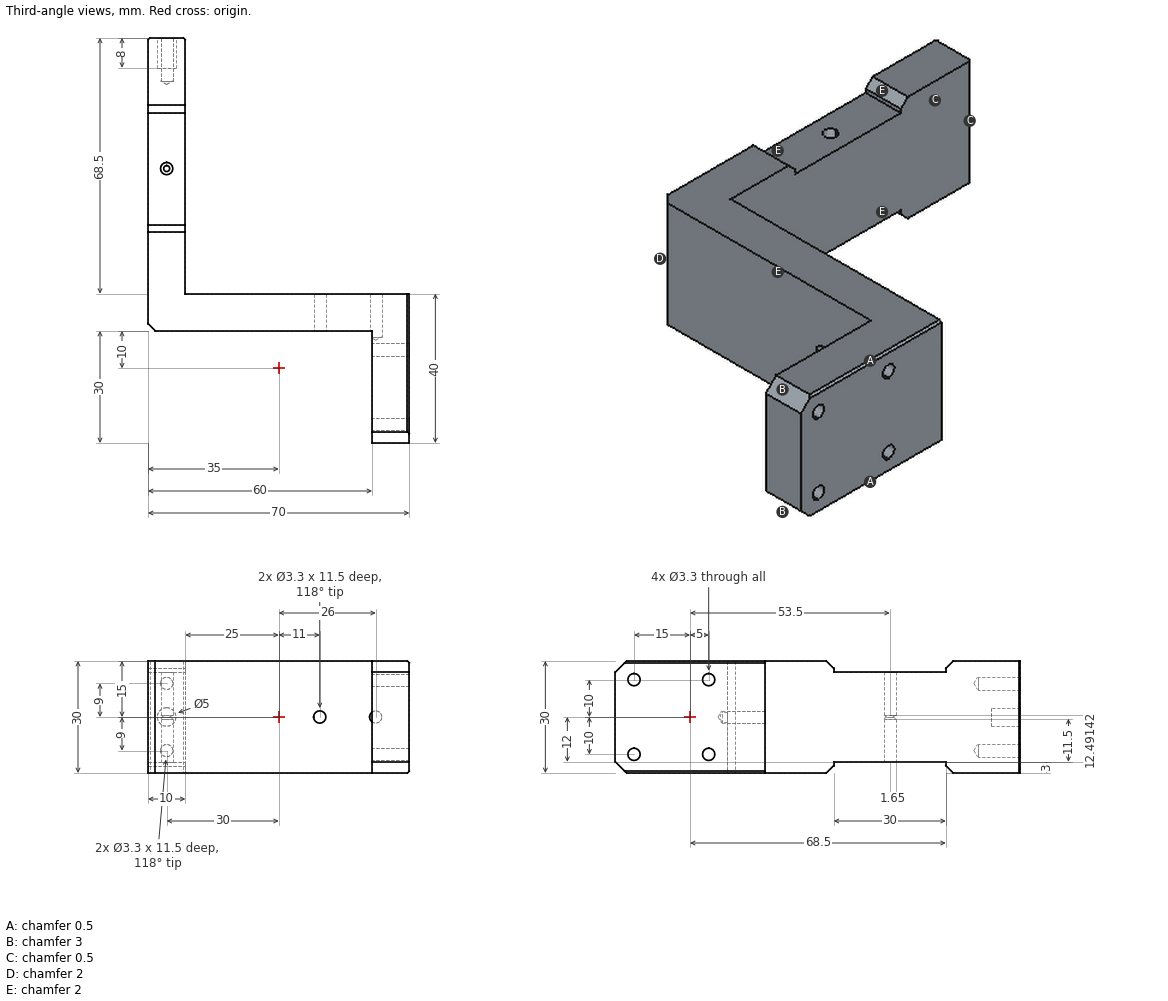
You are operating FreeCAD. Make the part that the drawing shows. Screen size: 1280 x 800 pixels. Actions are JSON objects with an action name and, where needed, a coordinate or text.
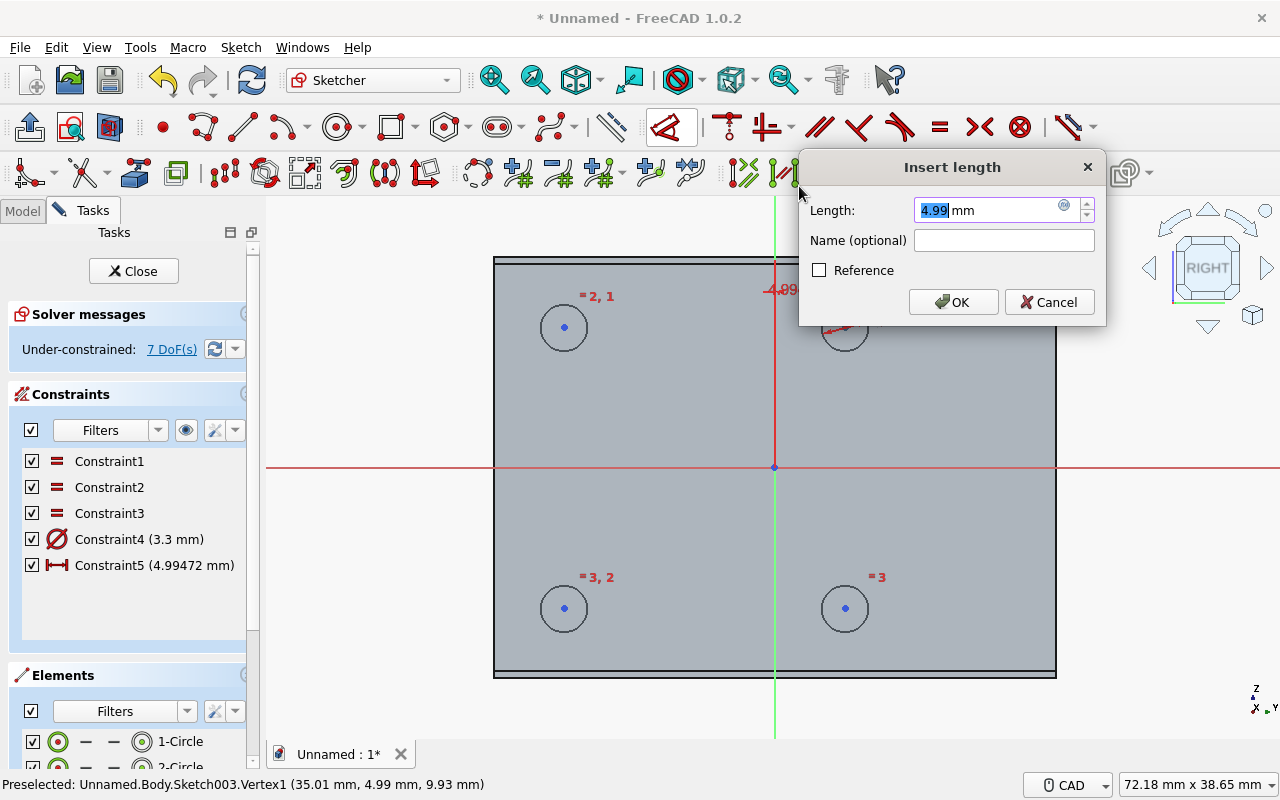
{"action": "type", "text": "5"}
{"action": "key", "text": "Return"}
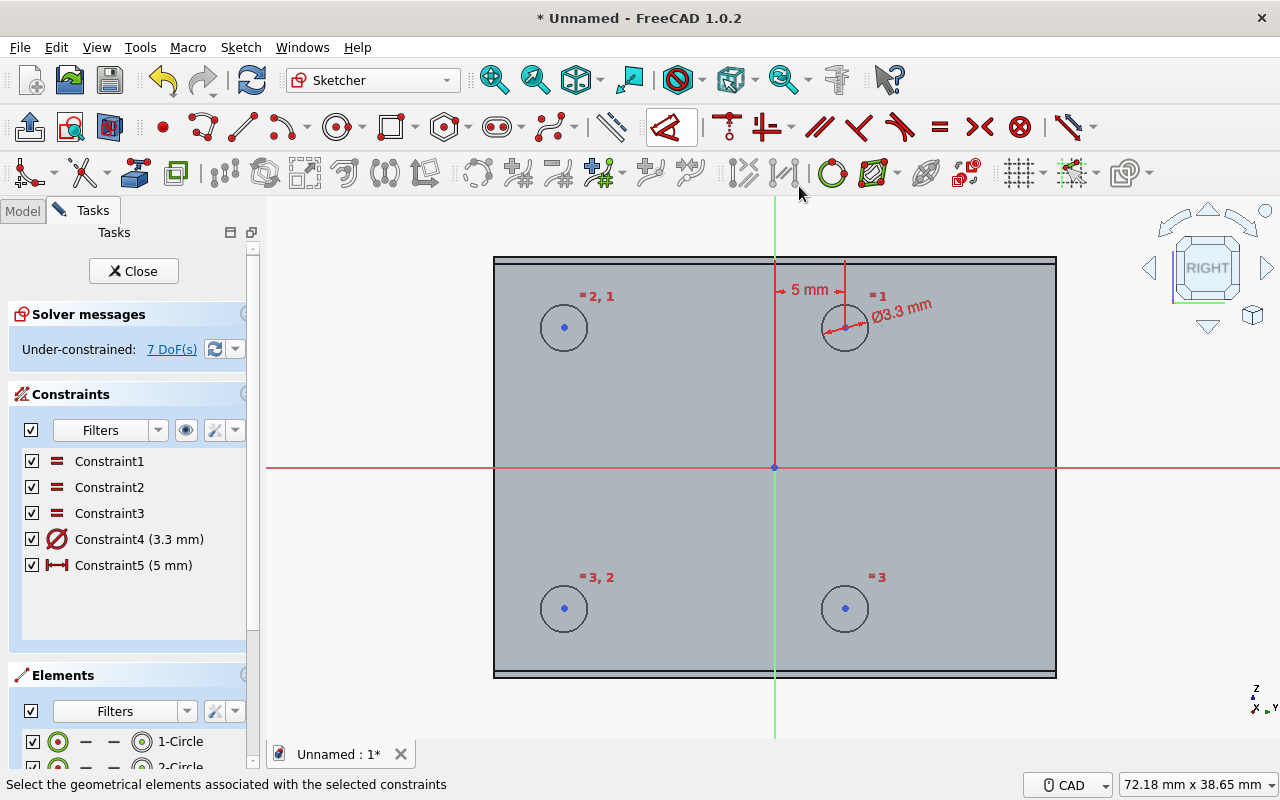
{"action": "left_click", "coordinate": [845, 609]}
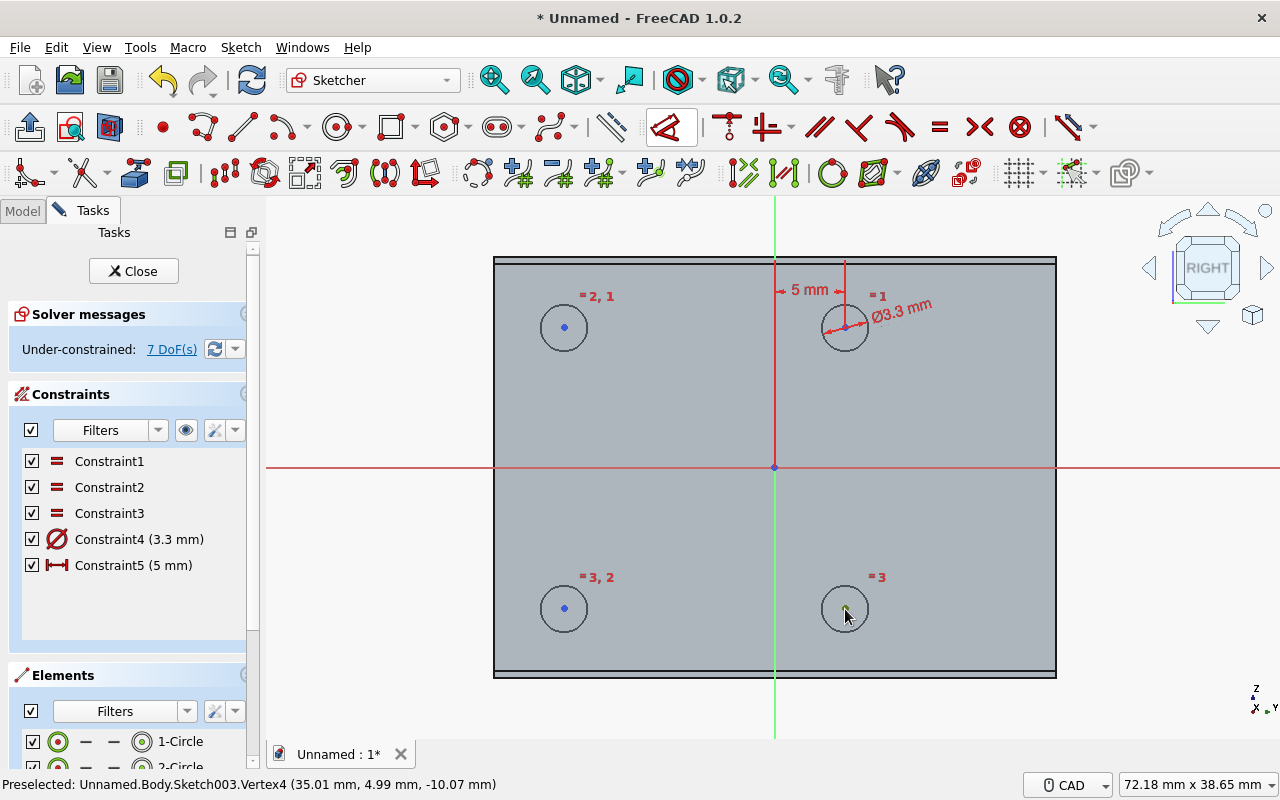
{"action": "left_click", "coordinate": [692, 128]}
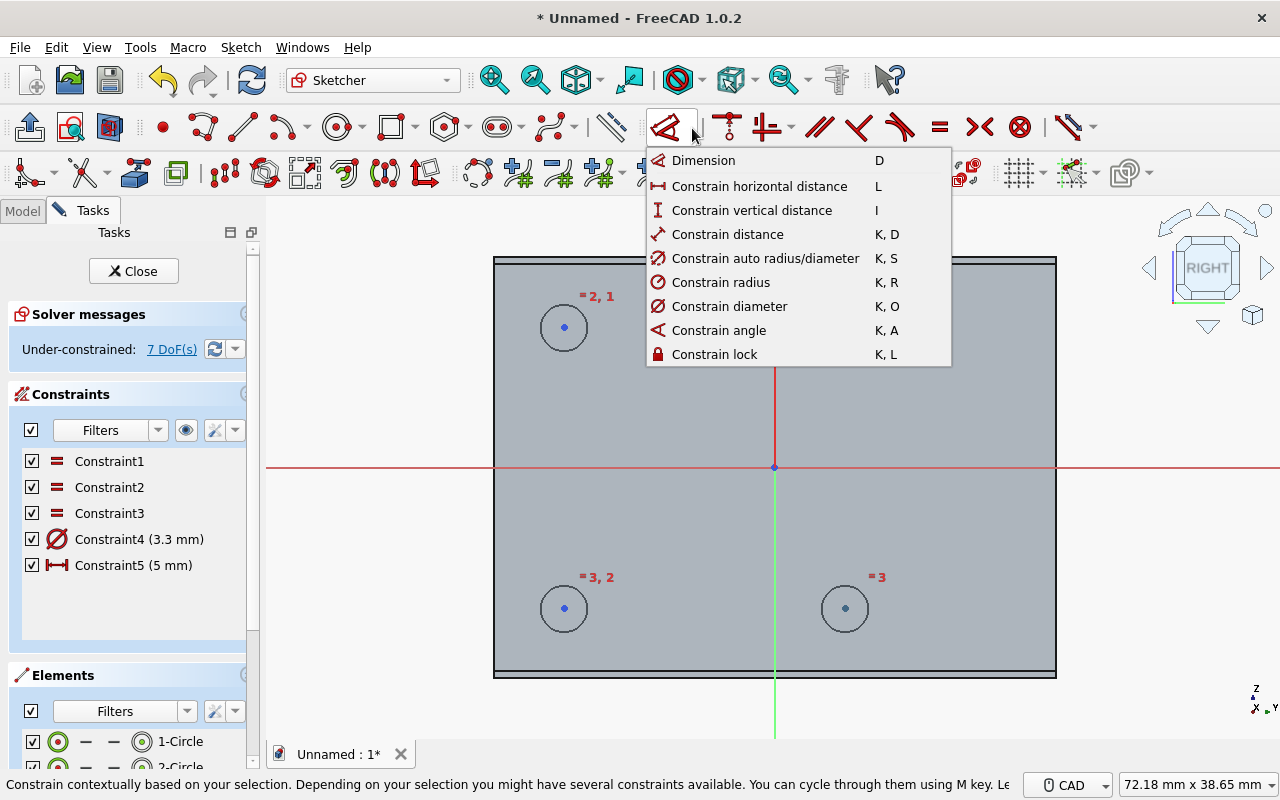
{"action": "left_click", "coordinate": [799, 186]}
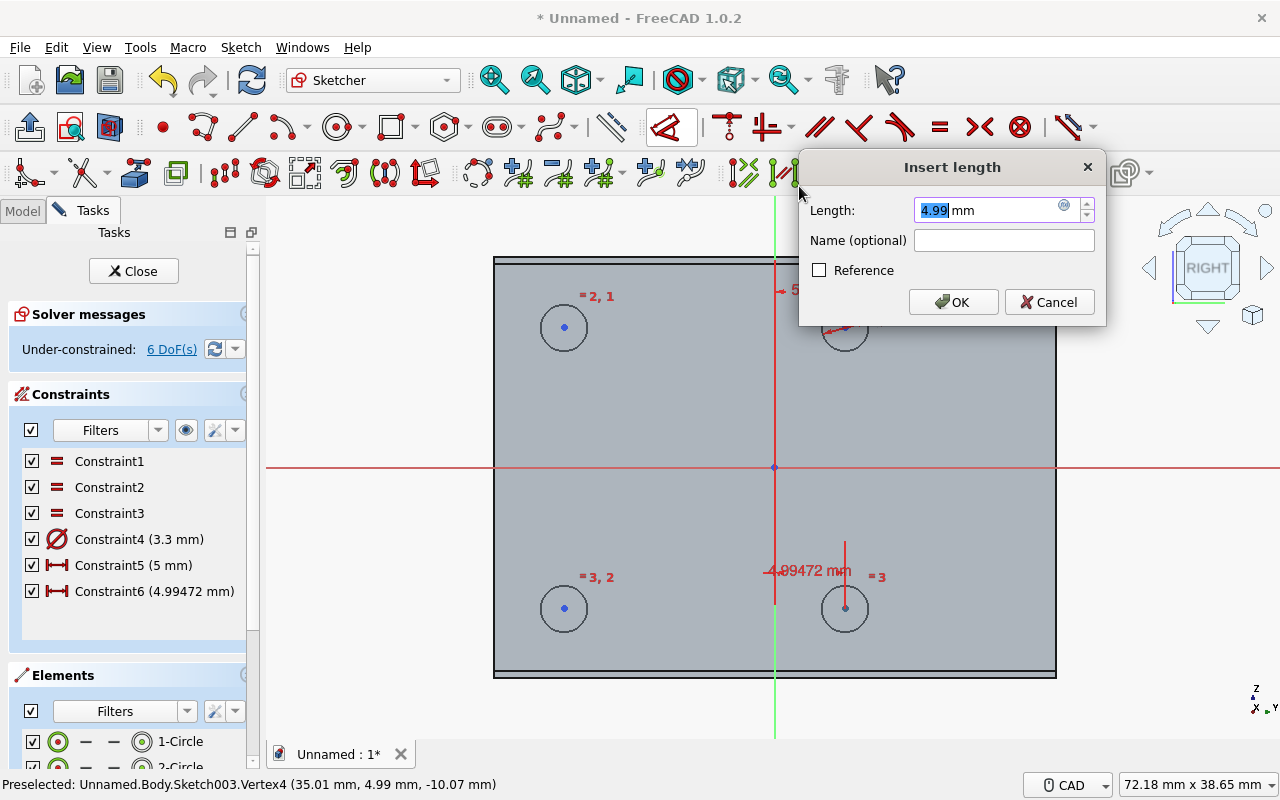
{"action": "type", "text": "5"}
{"action": "key", "text": "Return"}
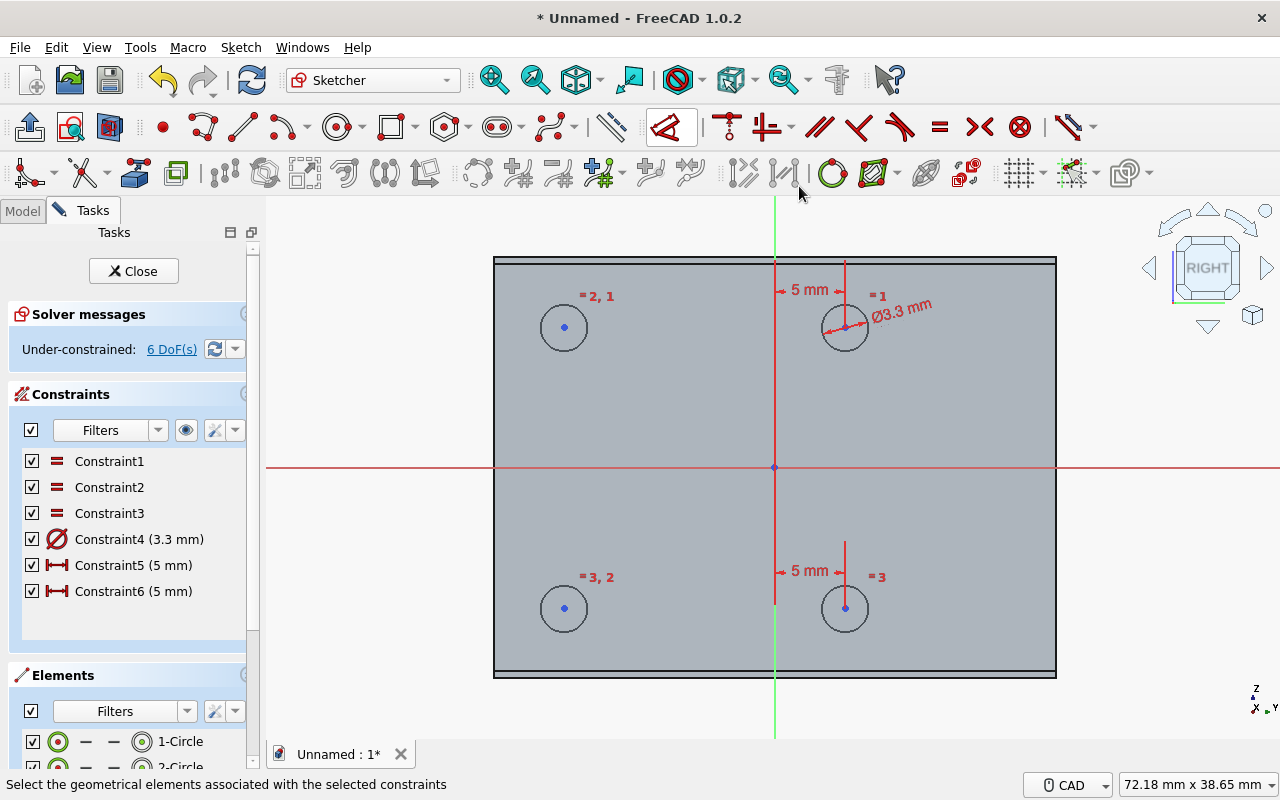
{"action": "left_click", "coordinate": [845, 328]}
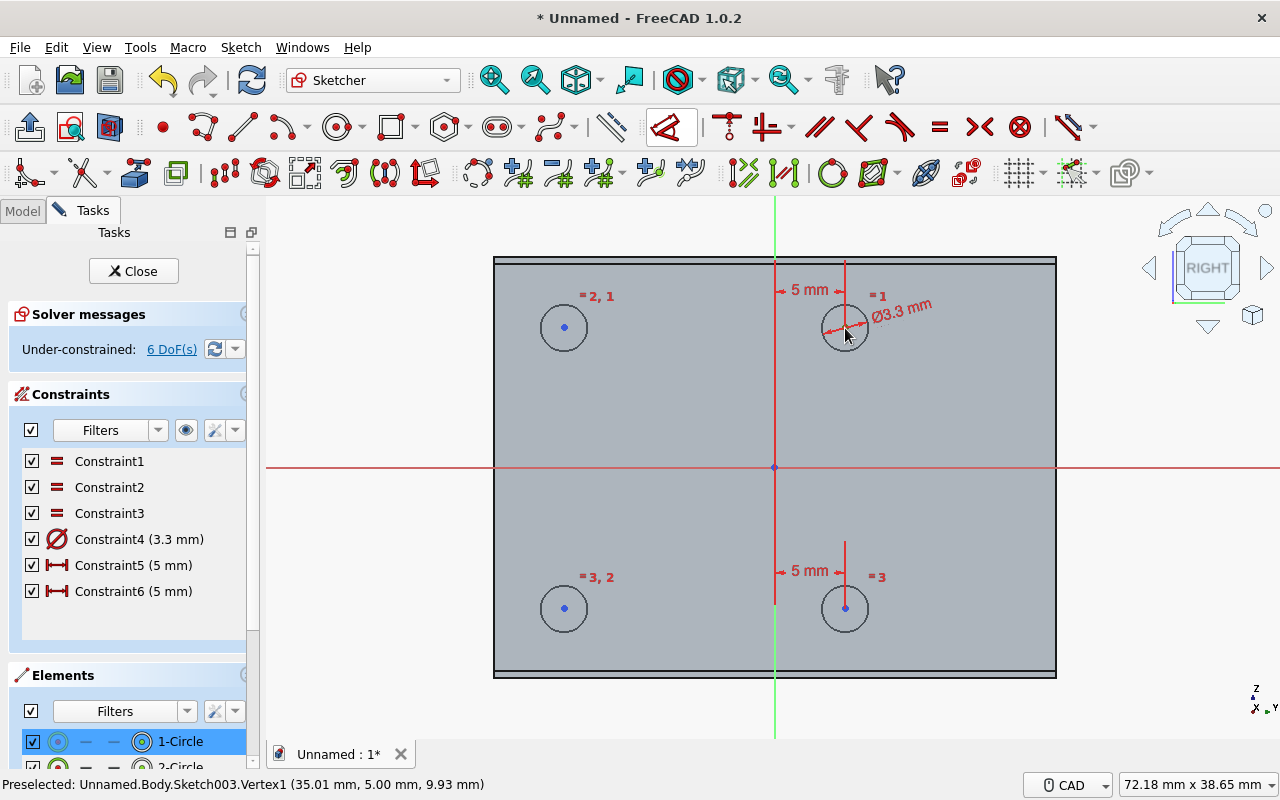
{"action": "key", "text": "i"}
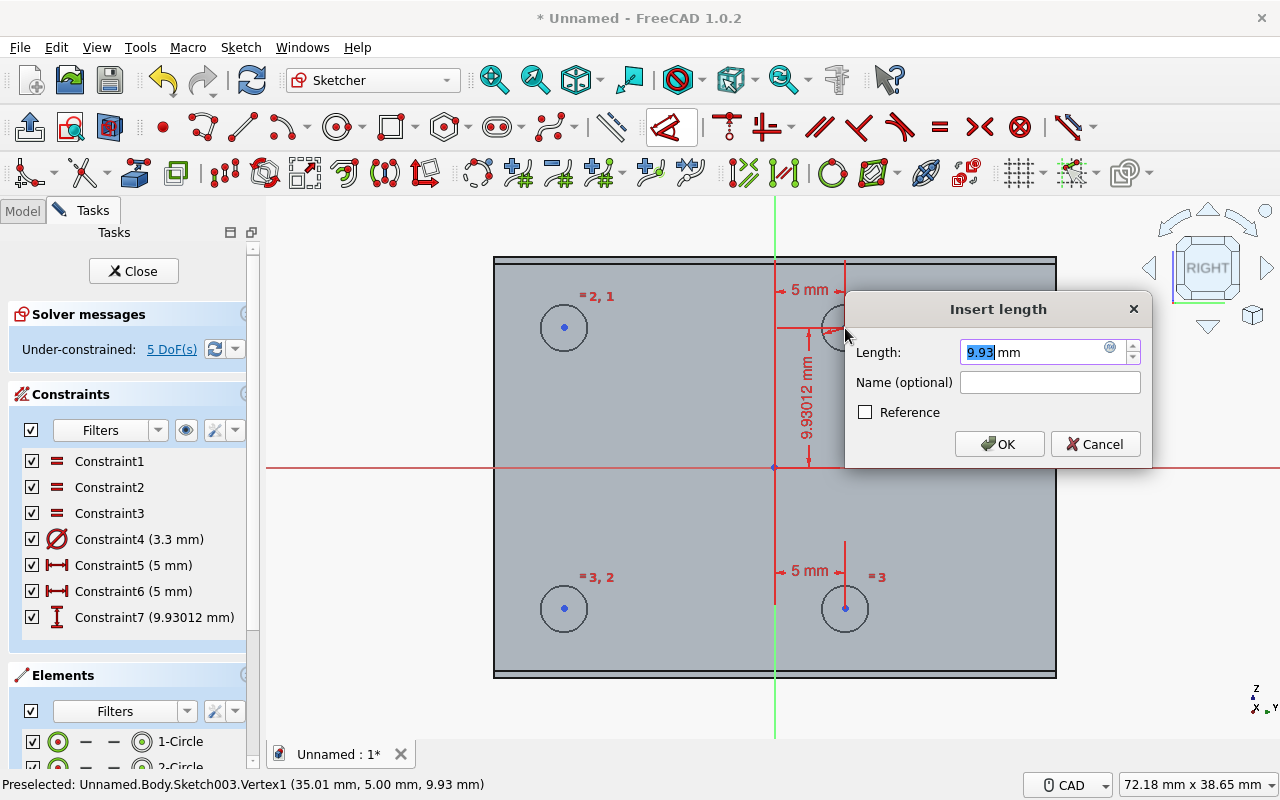
{"action": "type", "text": "10"}
{"action": "key", "text": "Return"}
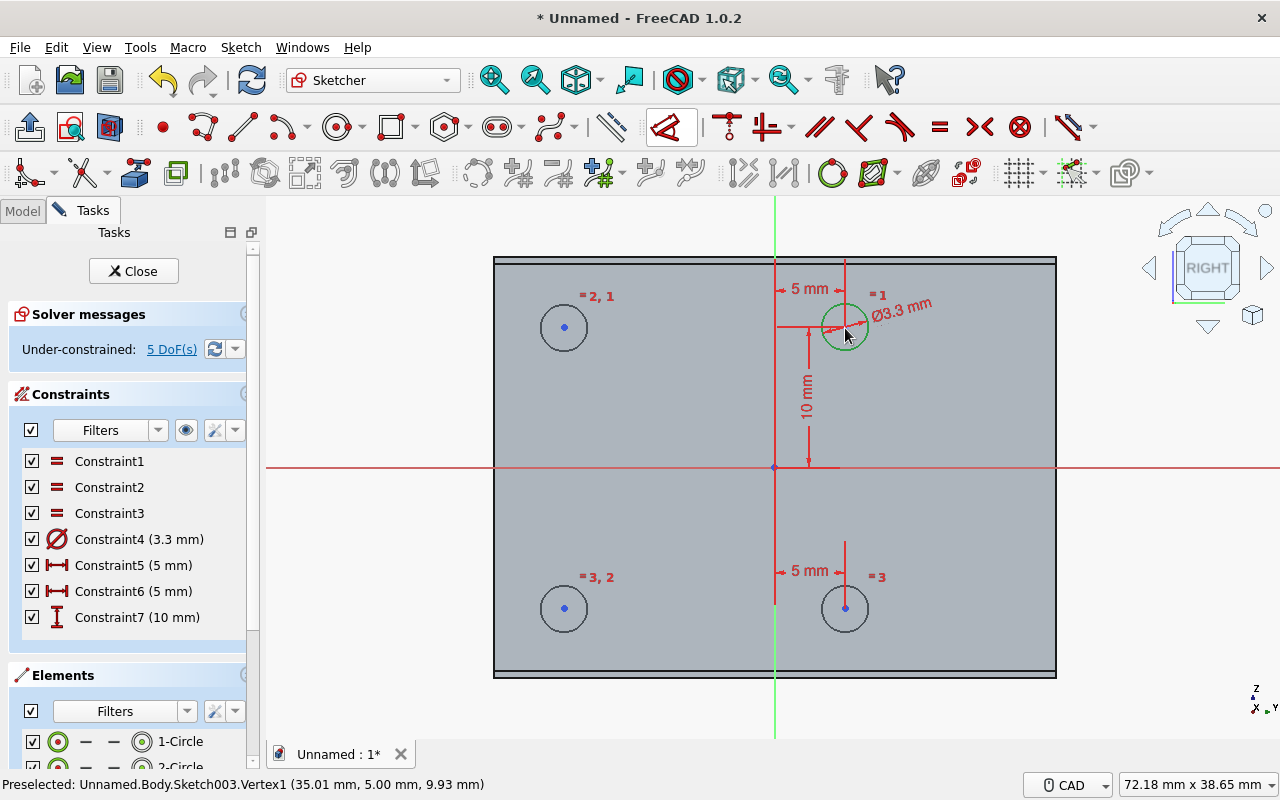
{"action": "left_click", "coordinate": [564, 328]}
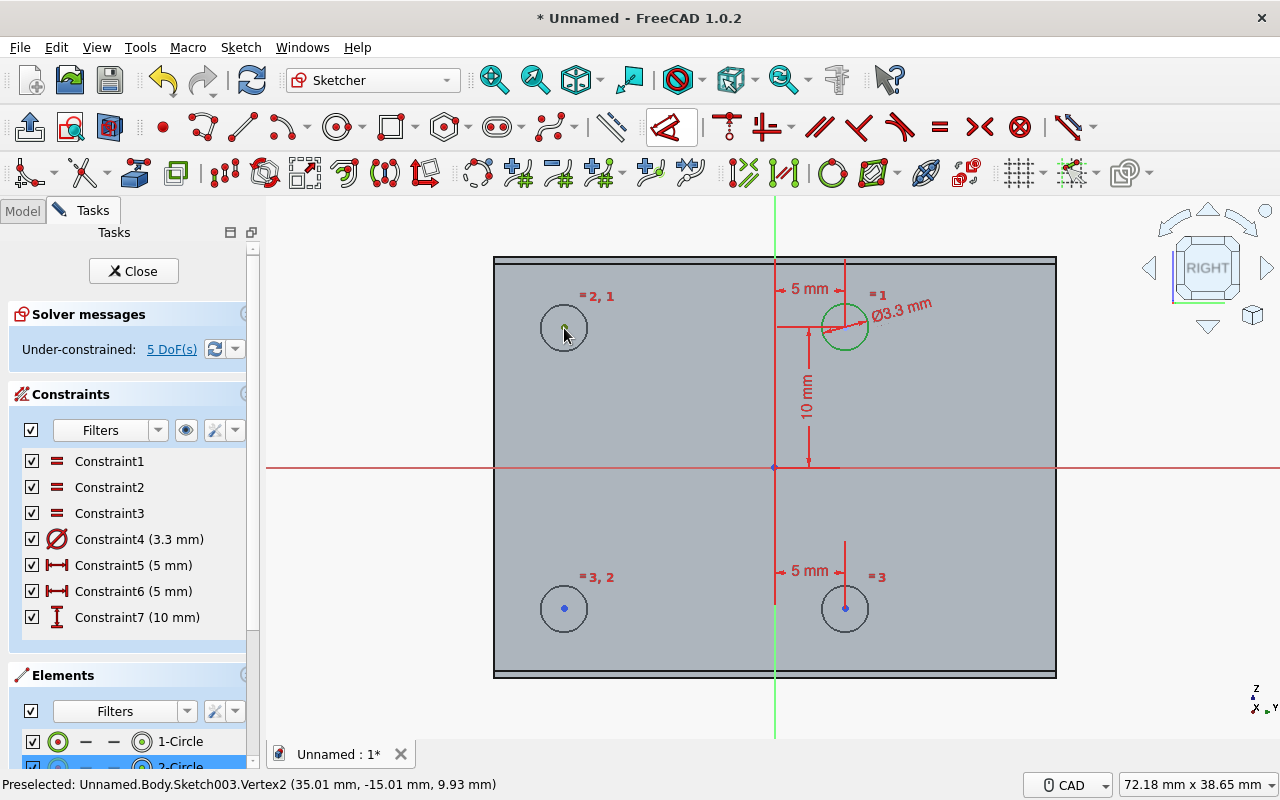
{"action": "left_click", "coordinate": [692, 128]}